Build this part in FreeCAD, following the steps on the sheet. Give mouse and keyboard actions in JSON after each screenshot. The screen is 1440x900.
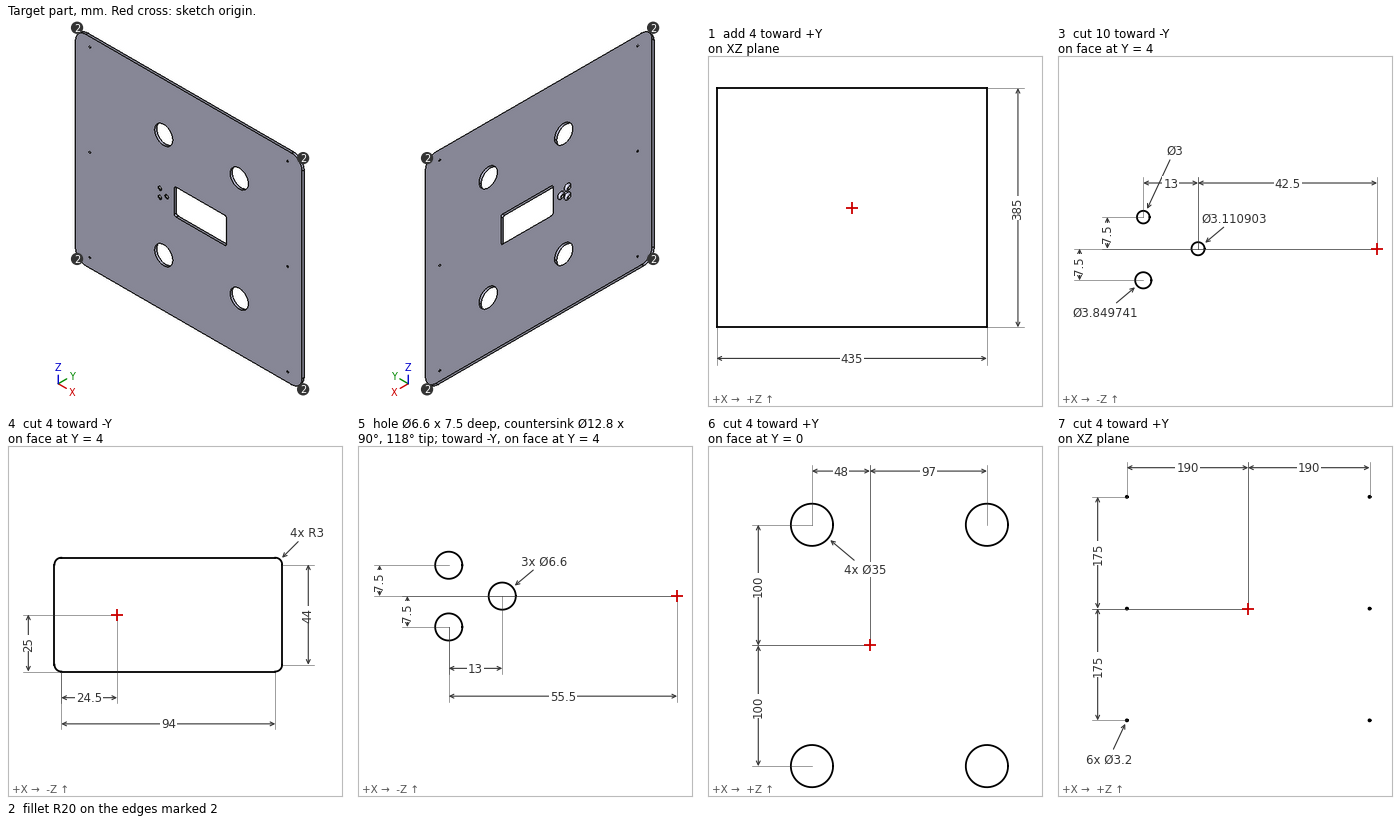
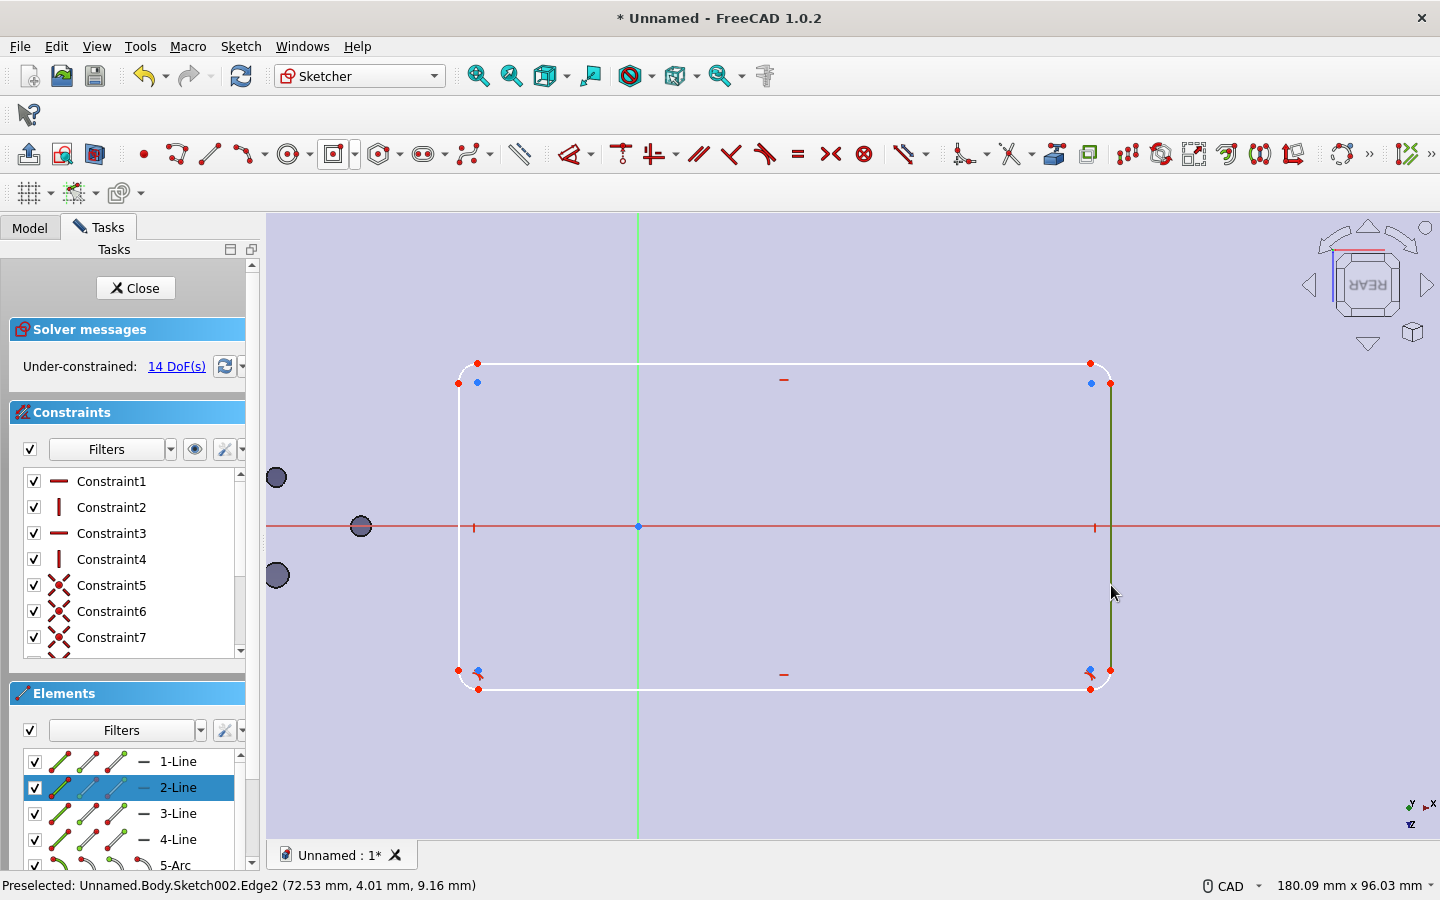
{"action": "scroll", "coordinate": [1099, 688], "scroll_direction": "up", "scroll_amount": 3}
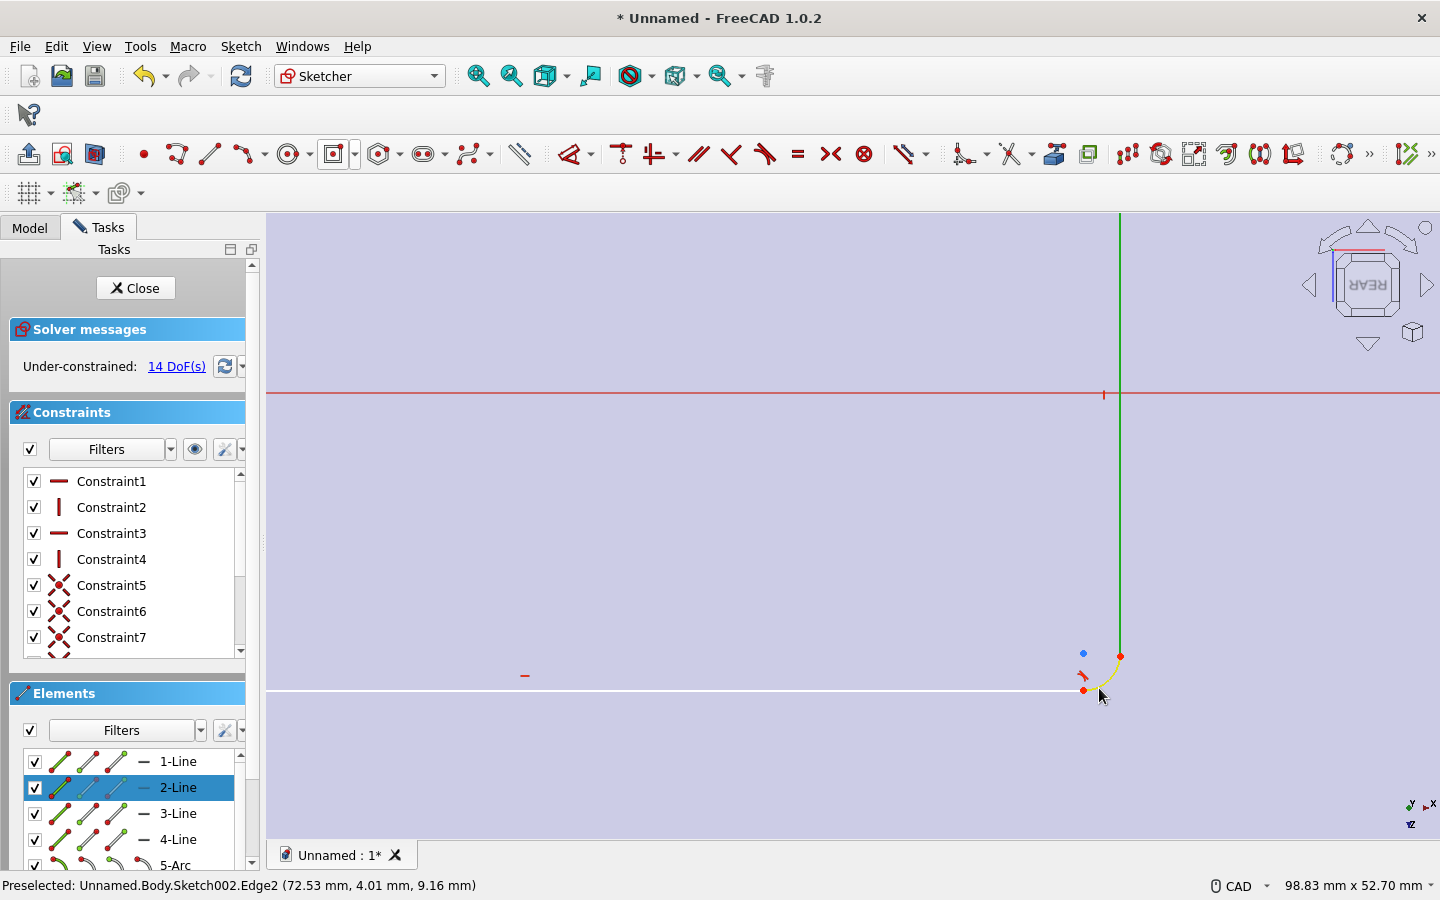
{"action": "left_click", "coordinate": [1099, 687]}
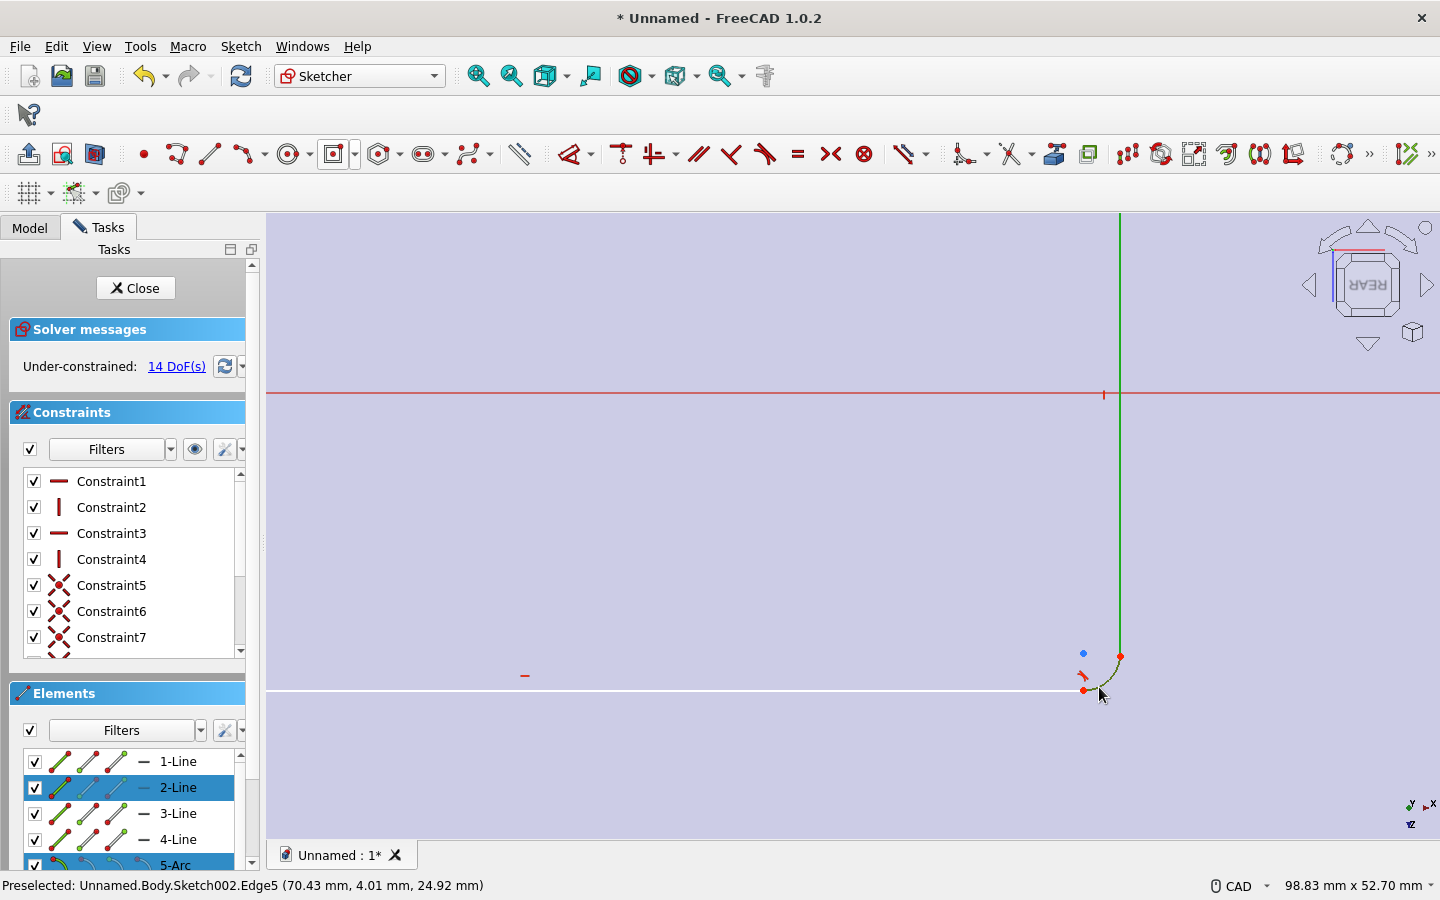
{"action": "left_click", "coordinate": [765, 154]}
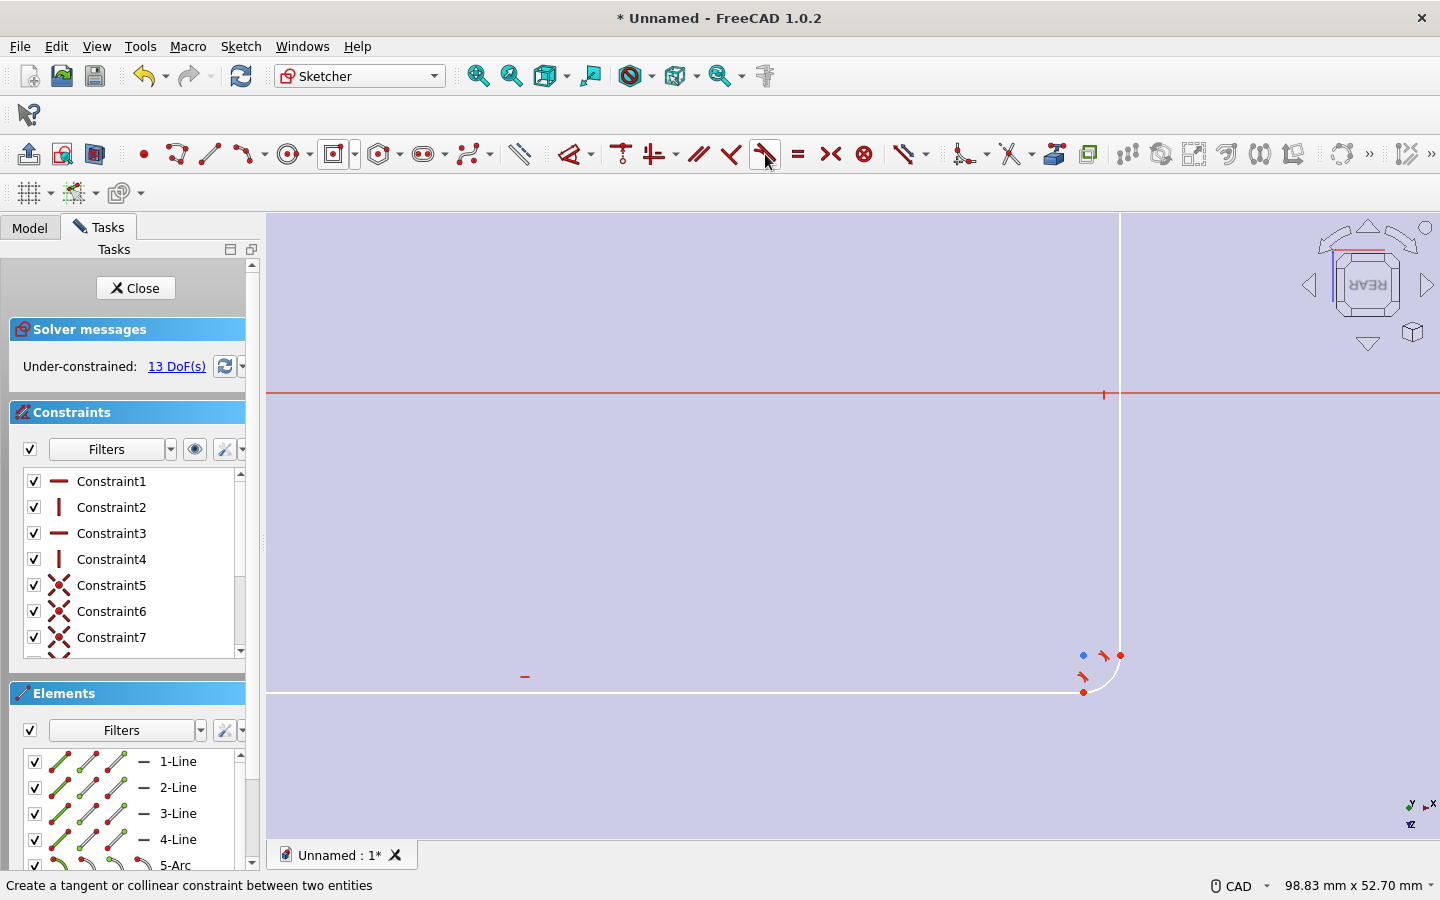
{"action": "left_click", "coordinate": [1120, 499]}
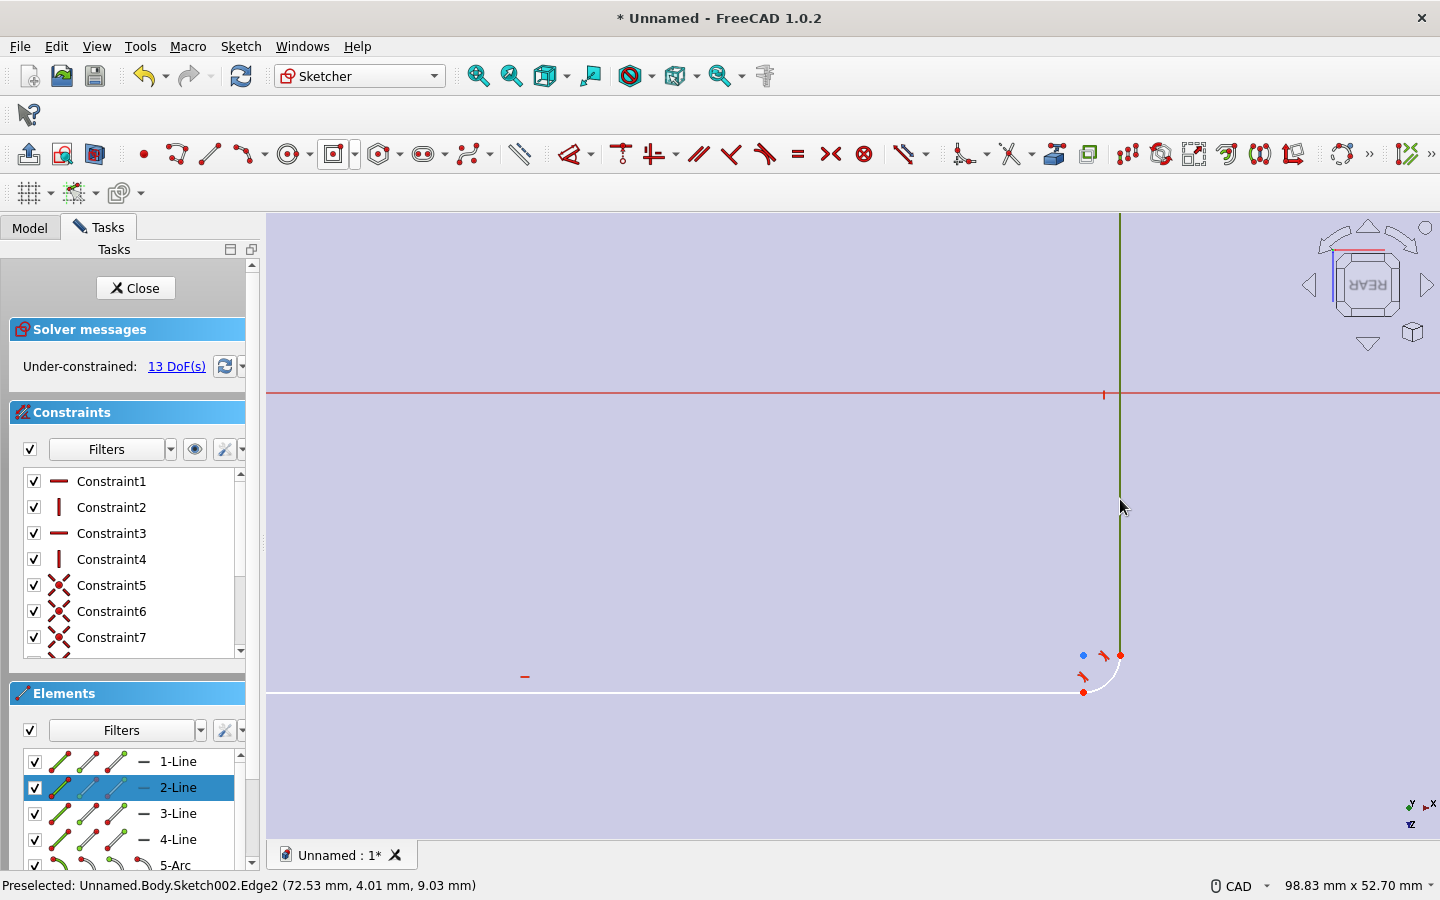
{"action": "scroll", "coordinate": [1099, 688], "scroll_direction": "down", "scroll_amount": 3}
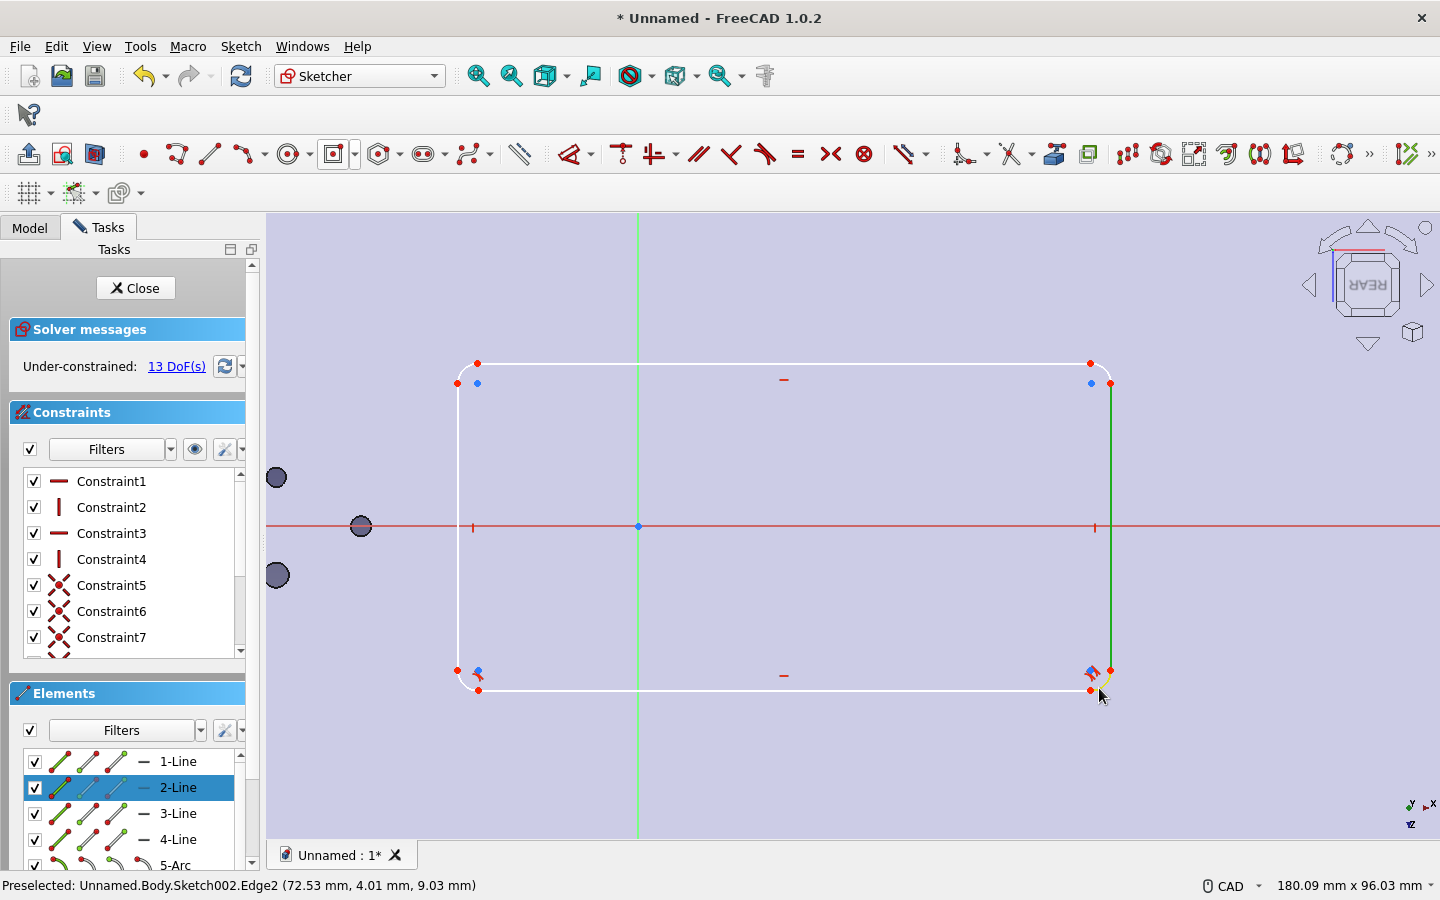
{"action": "scroll", "coordinate": [1109, 375], "scroll_direction": "up", "scroll_amount": 2}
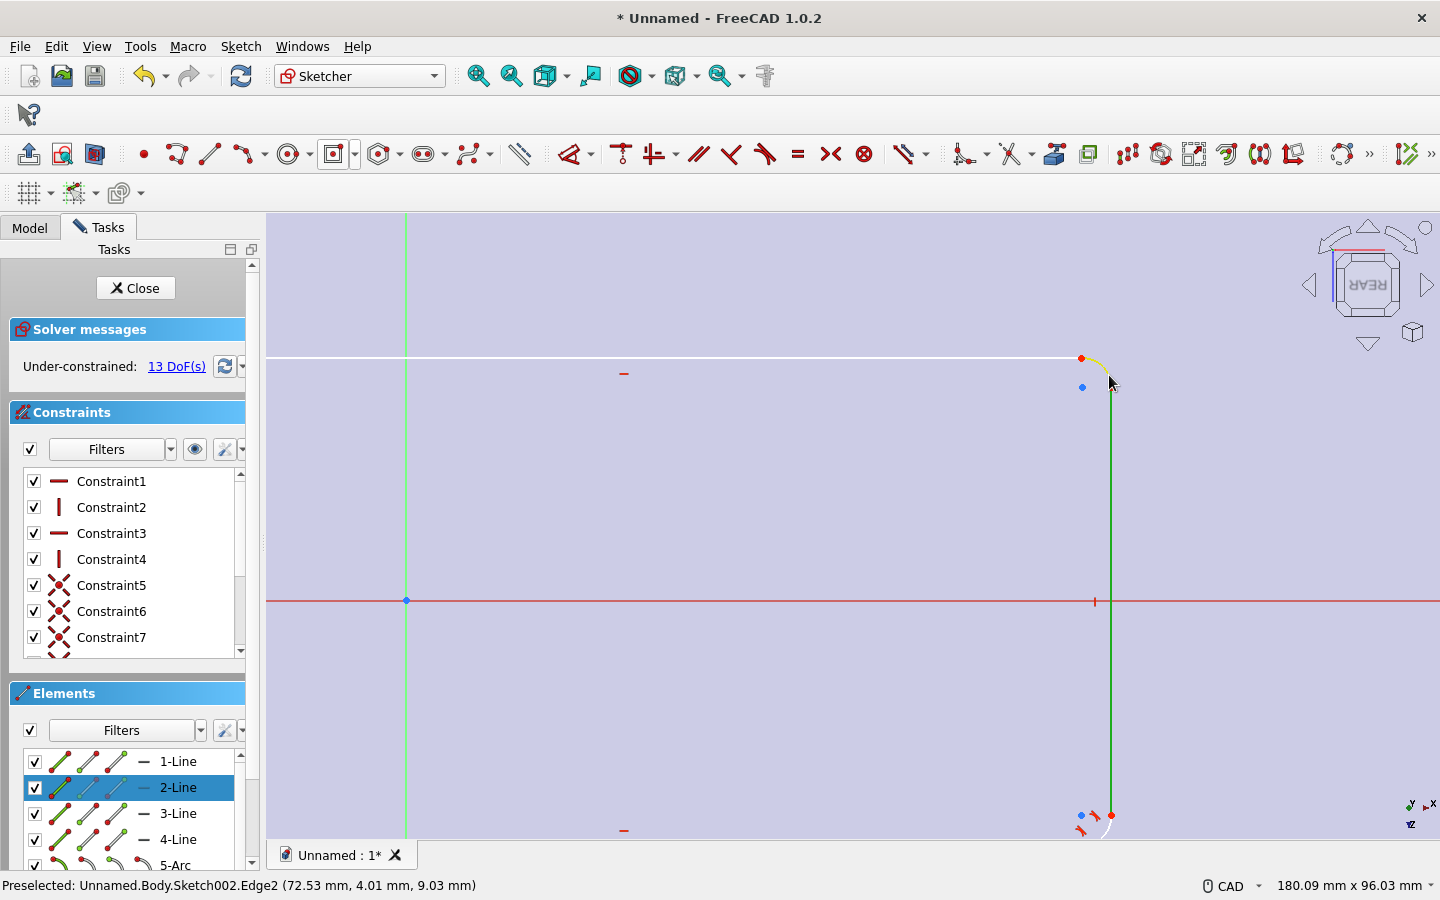
{"action": "left_click", "coordinate": [1108, 374]}